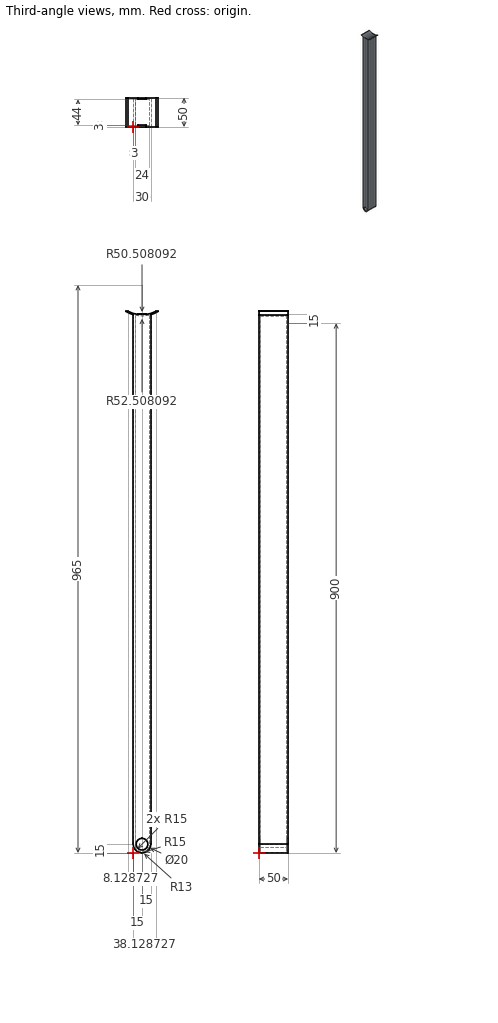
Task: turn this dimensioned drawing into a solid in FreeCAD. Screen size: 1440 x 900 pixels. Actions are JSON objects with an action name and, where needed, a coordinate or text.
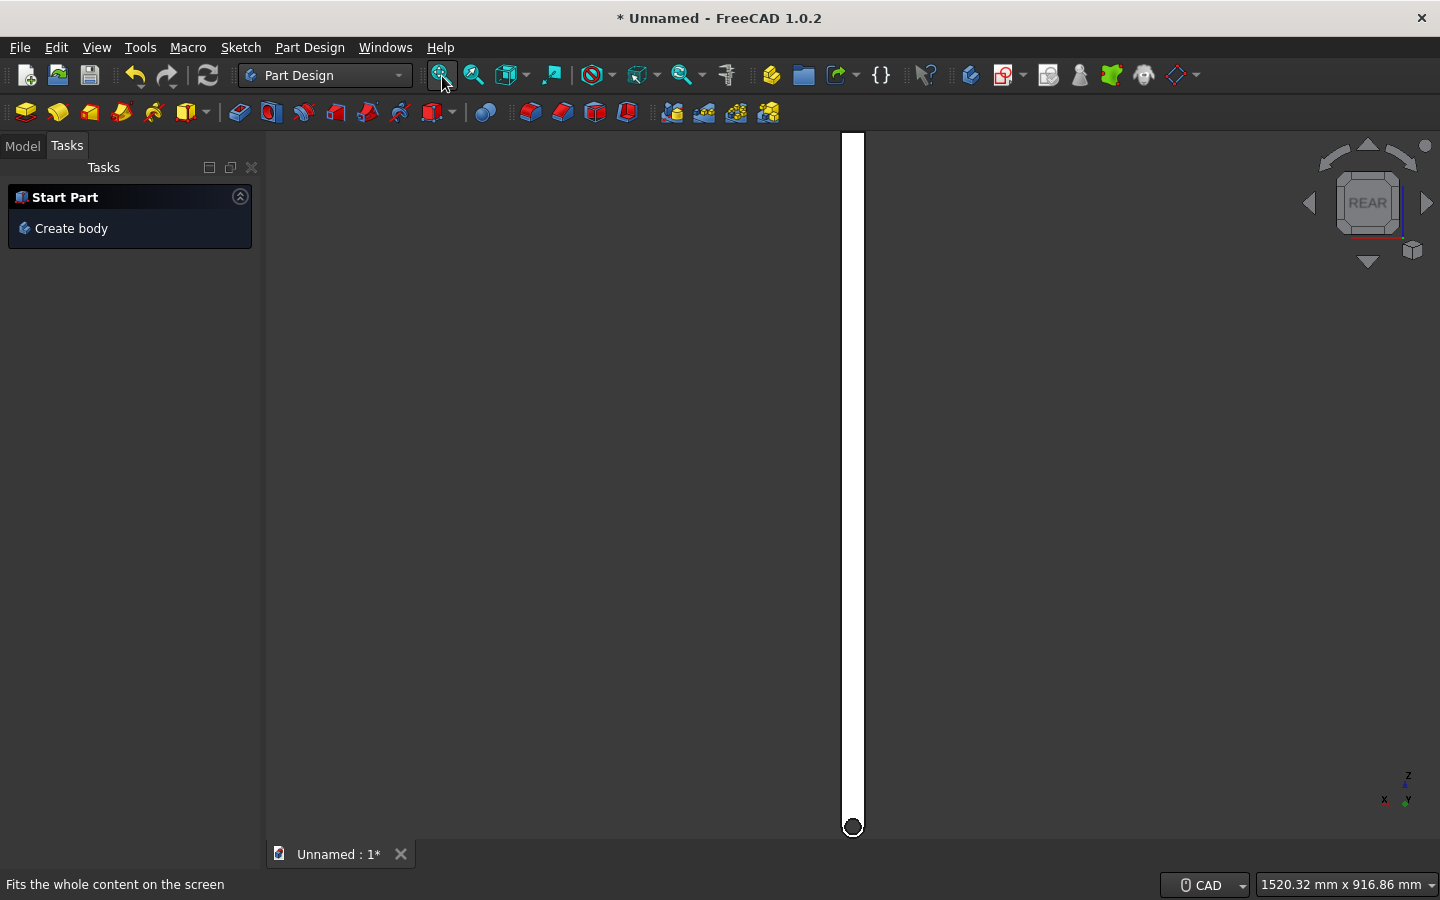
{"action": "left_click", "coordinate": [853, 181]}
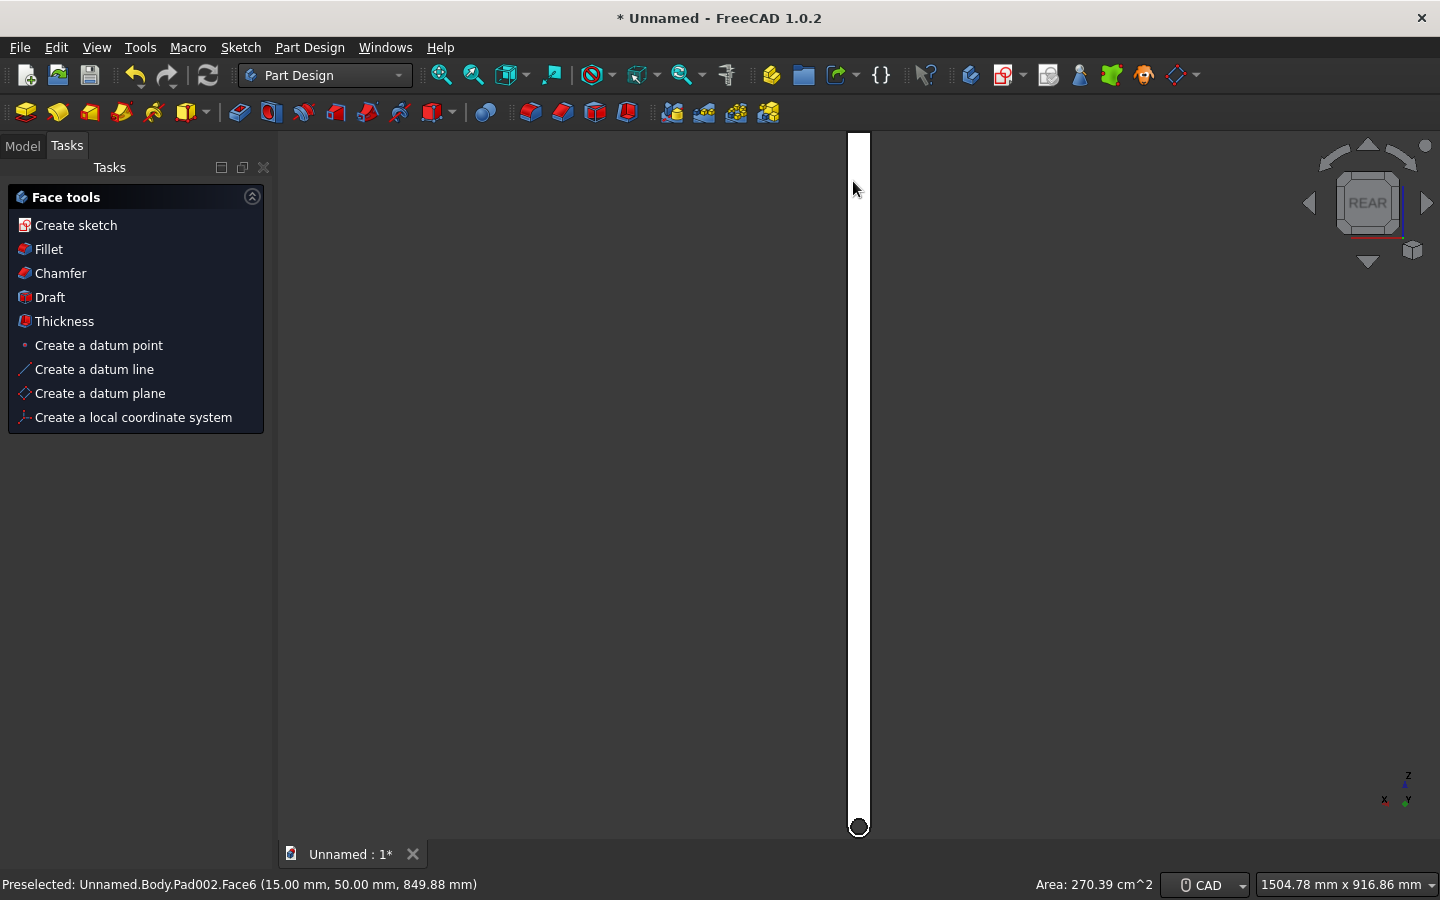
{"action": "left_click", "coordinate": [1004, 76]}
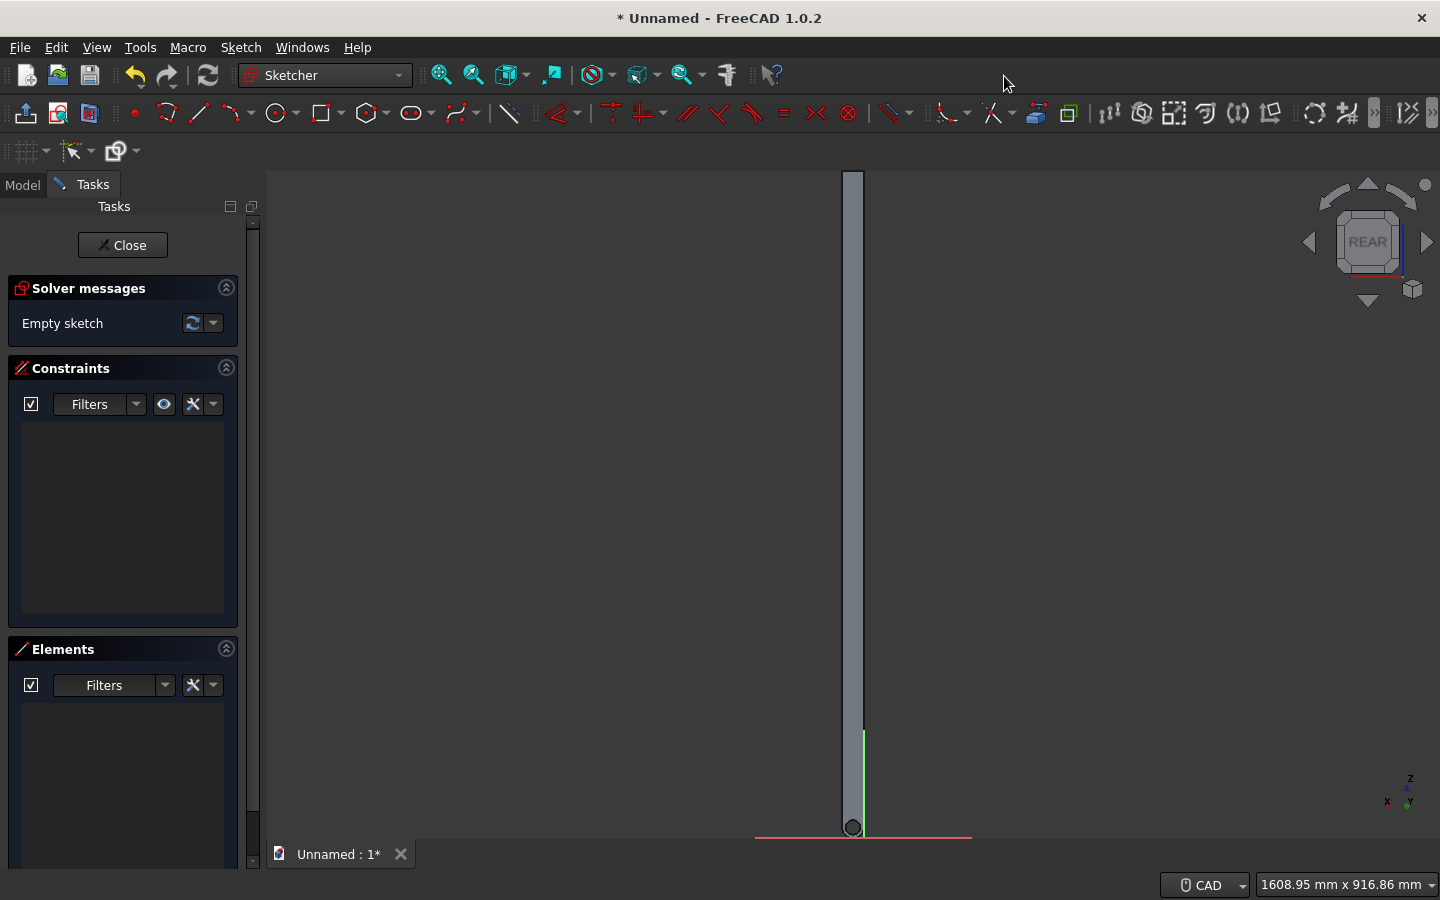
{"action": "scroll", "coordinate": [784, 504], "scroll_direction": "down", "scroll_amount": 5}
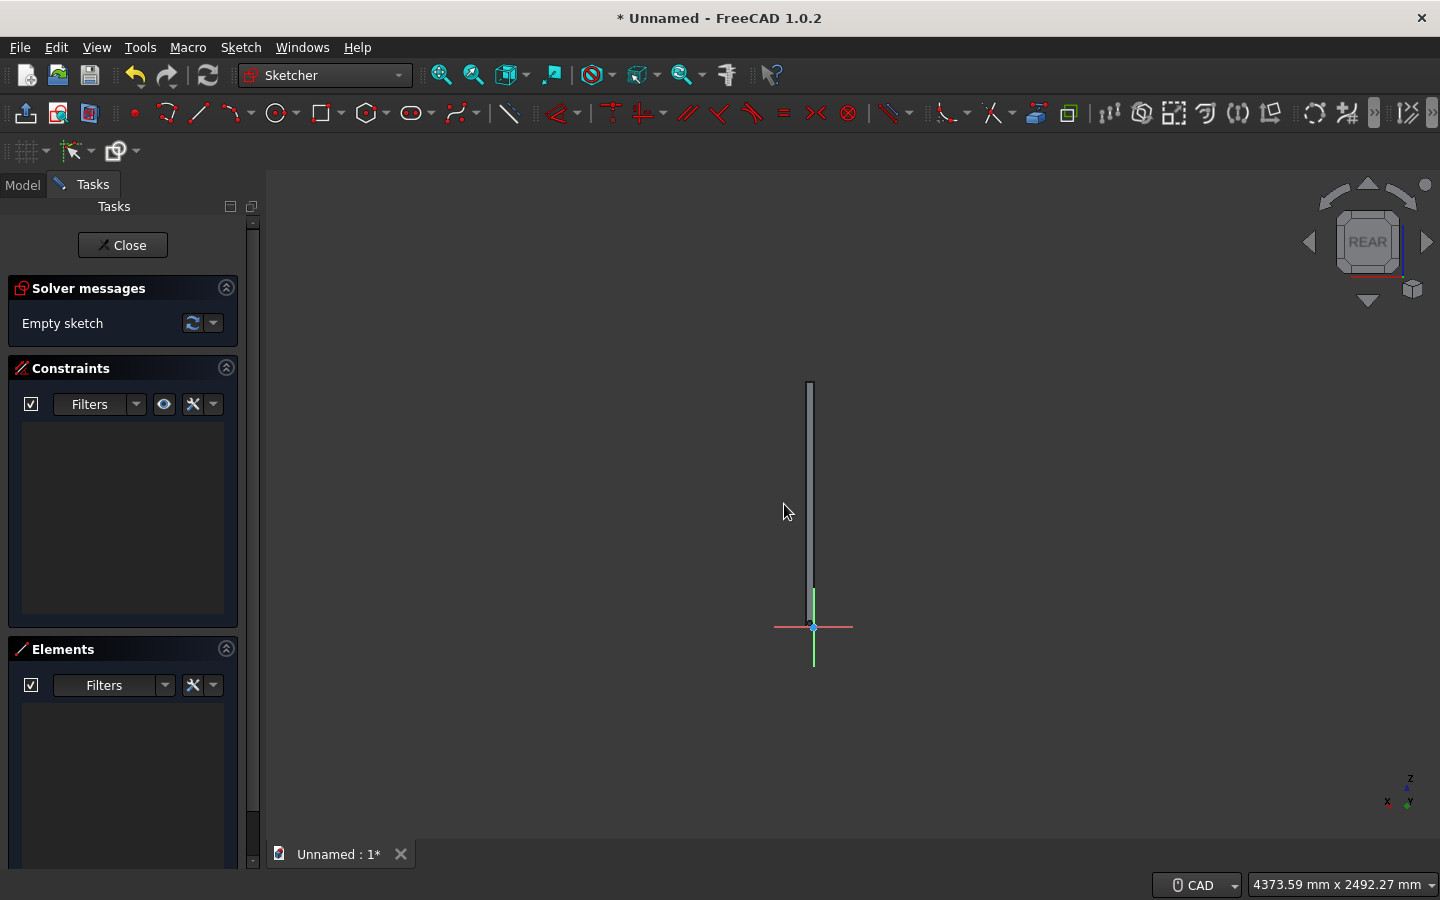
{"action": "scroll", "coordinate": [811, 375], "scroll_direction": "up", "scroll_amount": 15}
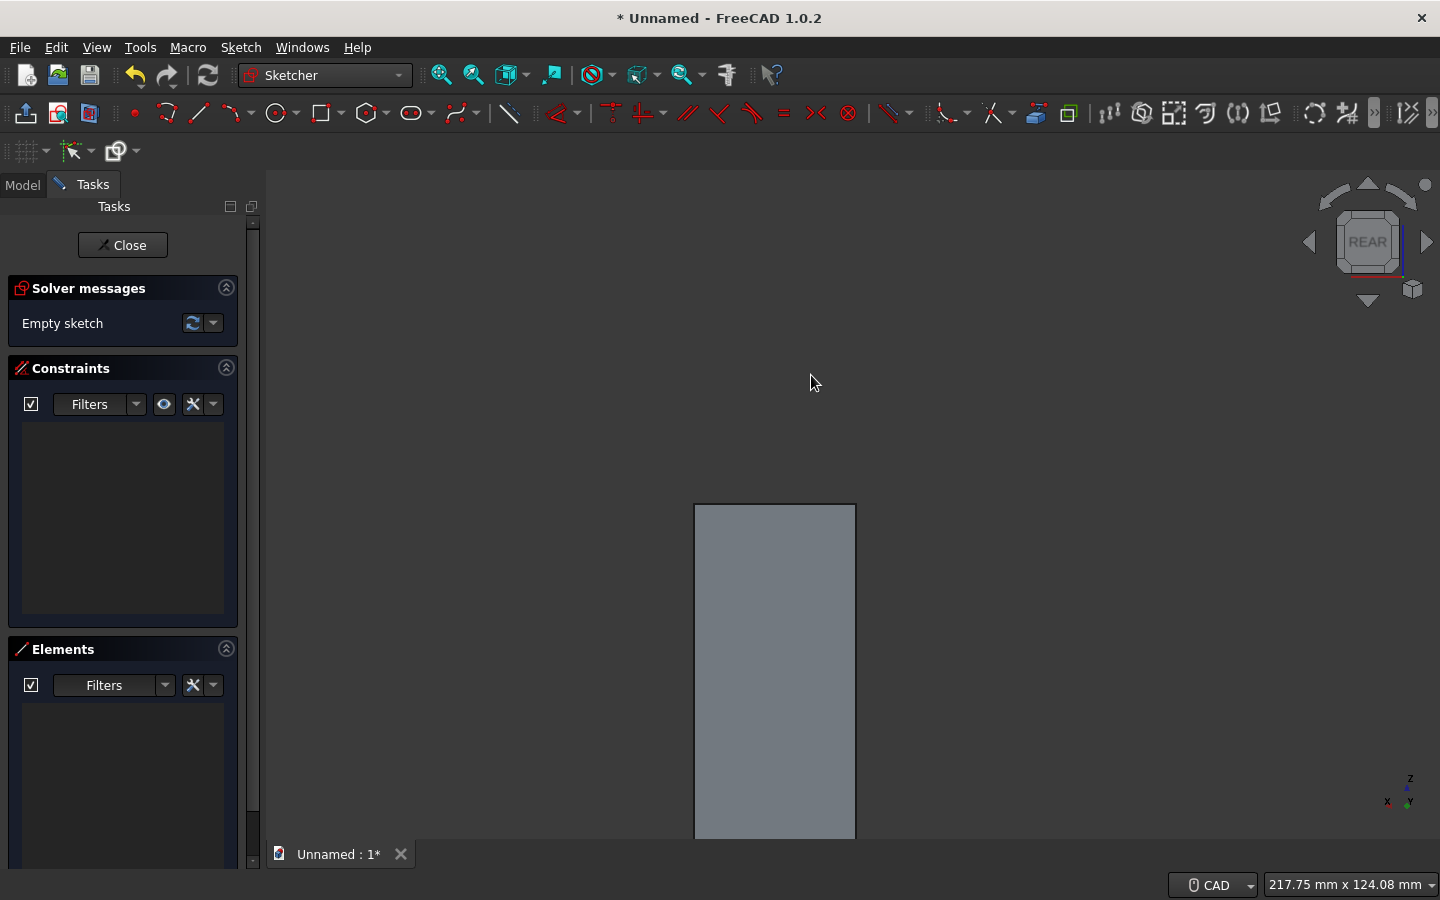
{"action": "scroll", "coordinate": [768, 490], "scroll_direction": "up", "scroll_amount": 4}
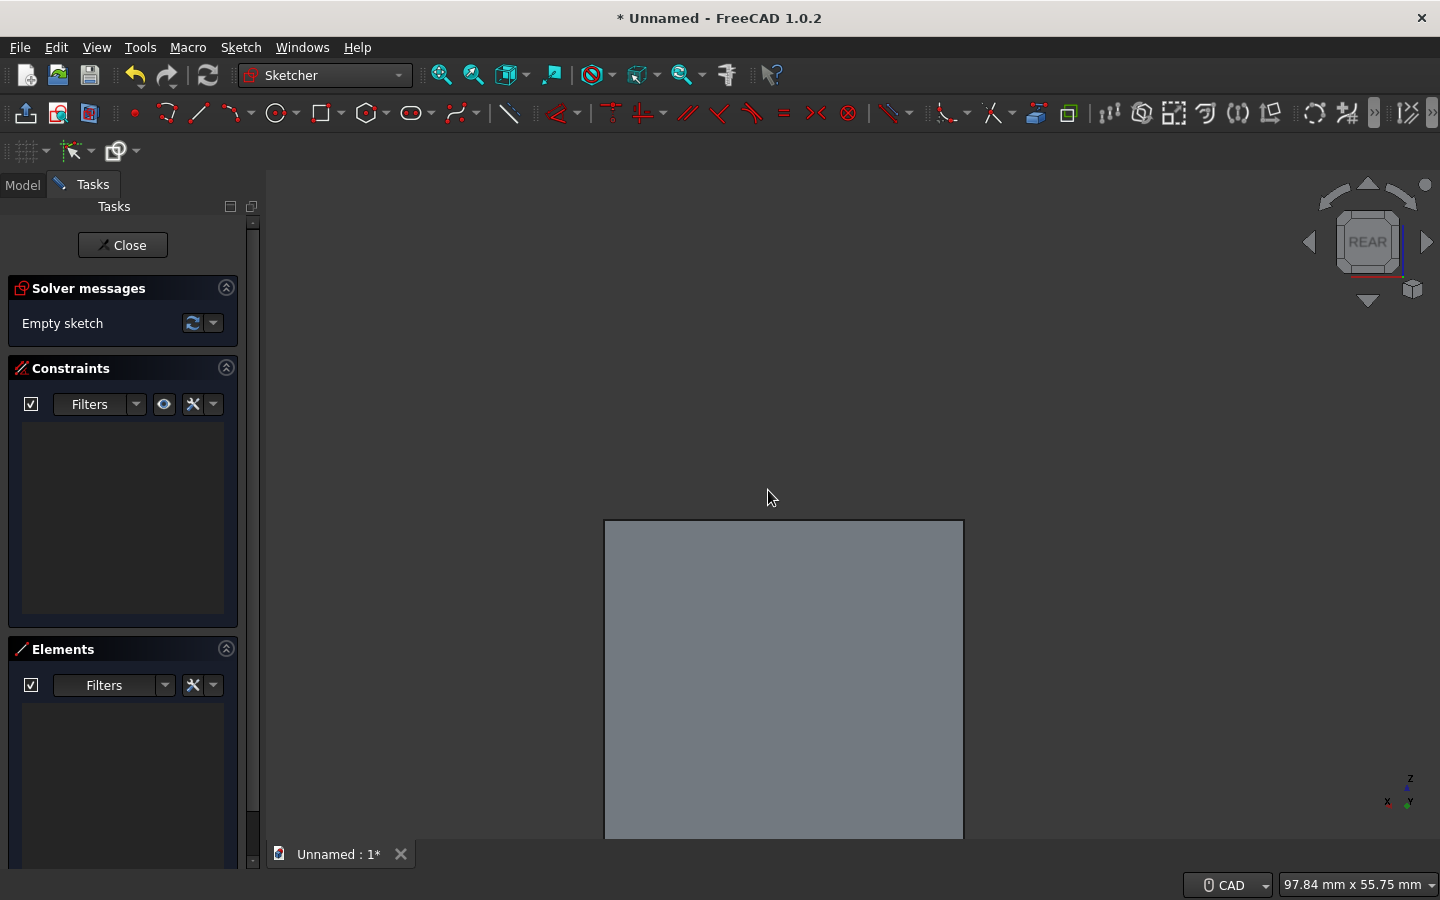
{"action": "left_click", "coordinate": [200, 114]}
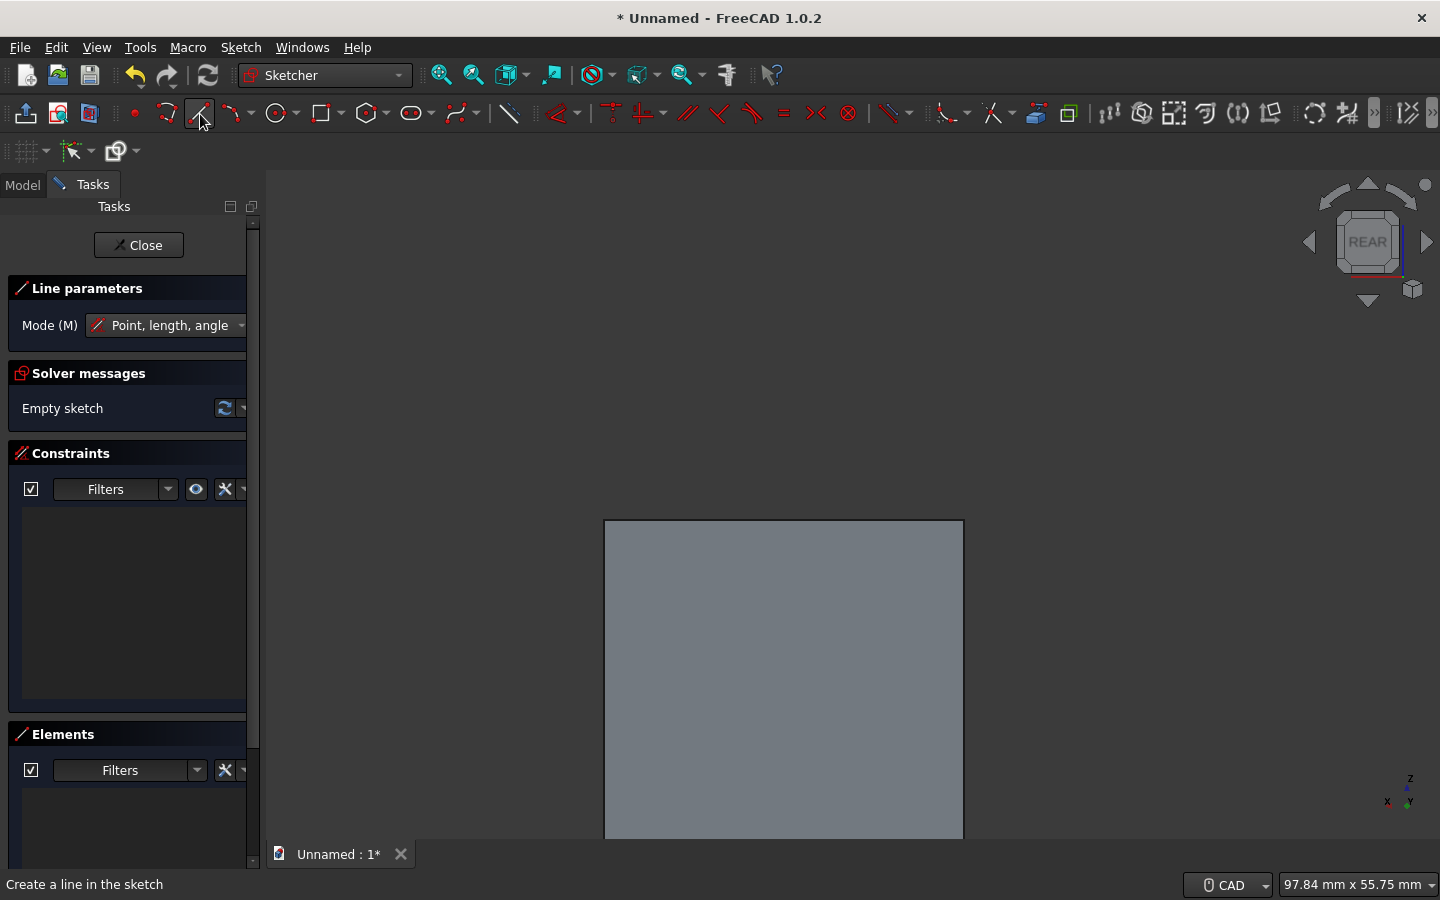
{"action": "left_click", "coordinate": [1110, 458]}
{"action": "left_click", "coordinate": [1061, 458]}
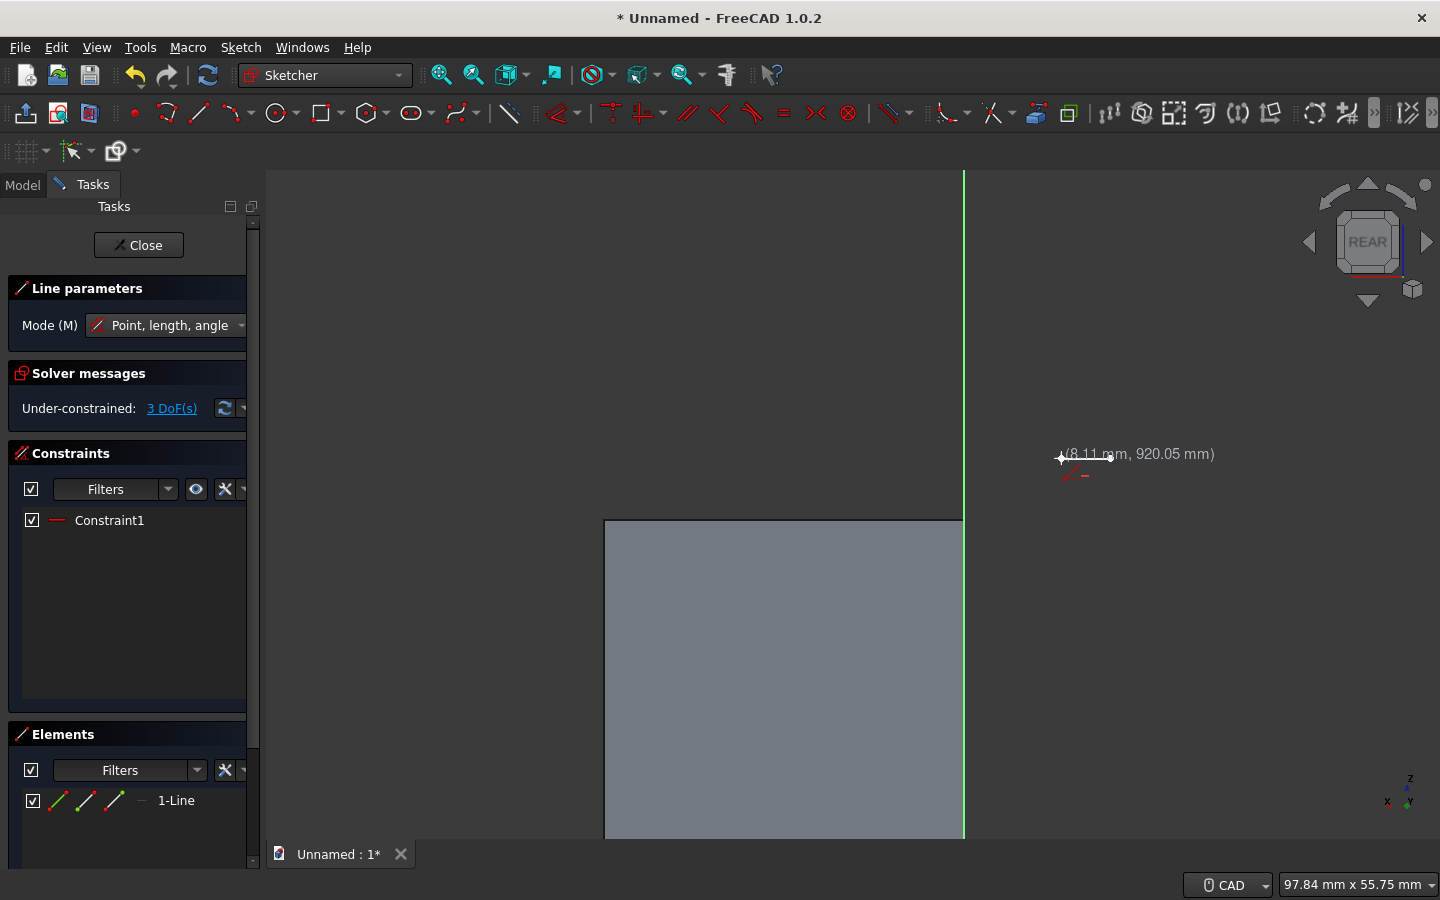
{"action": "left_click", "coordinate": [506, 458]}
{"action": "left_click", "coordinate": [457, 458]}